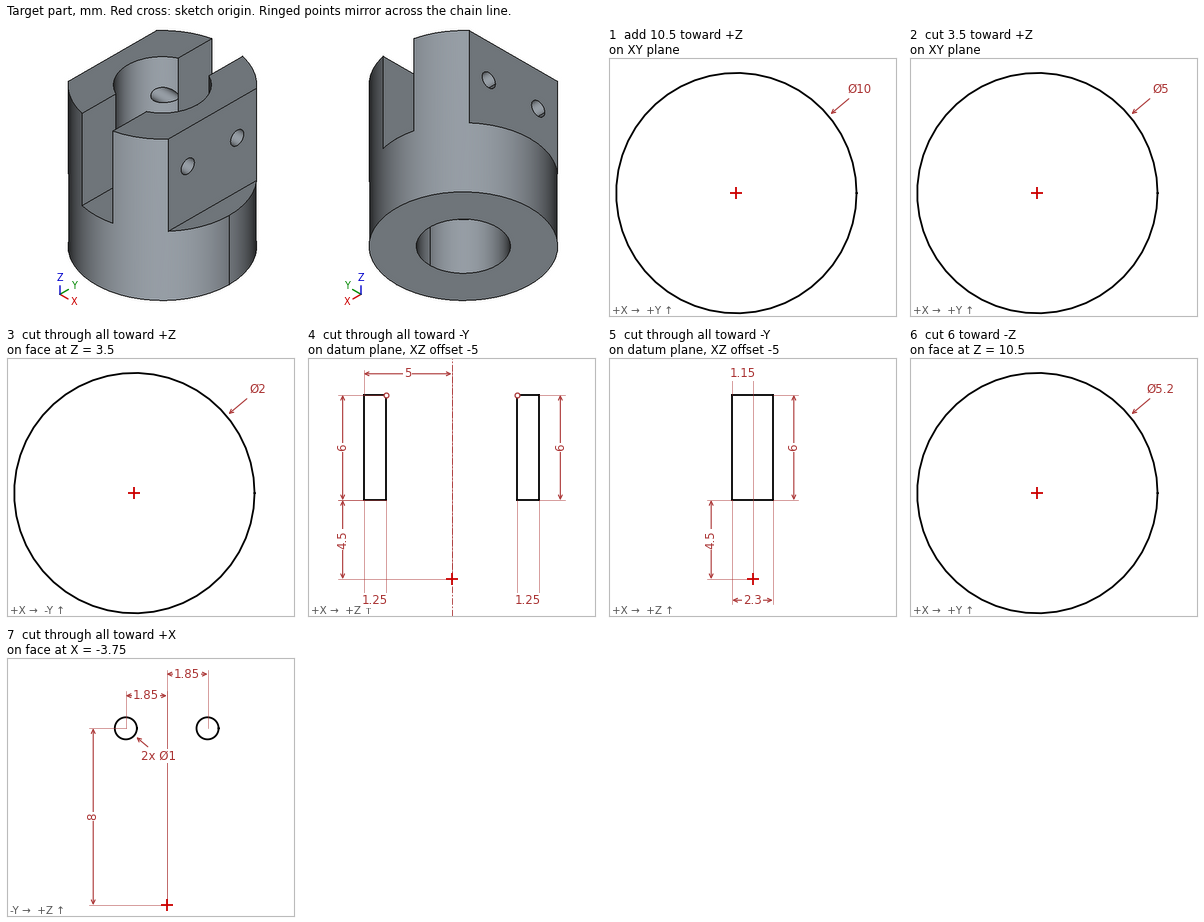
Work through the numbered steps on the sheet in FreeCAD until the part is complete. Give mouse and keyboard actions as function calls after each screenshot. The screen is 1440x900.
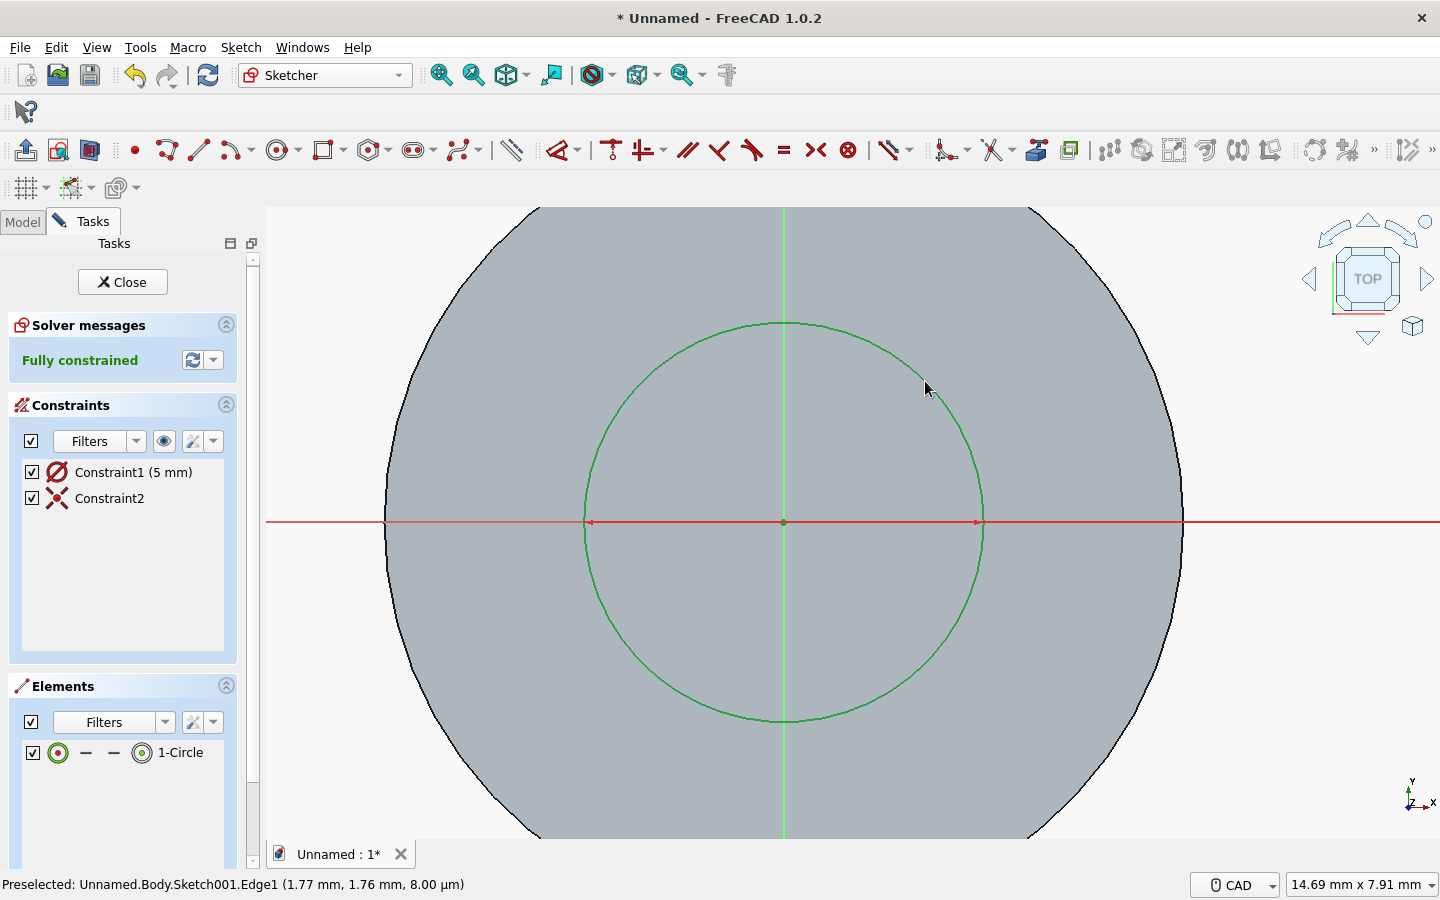
click(123, 282)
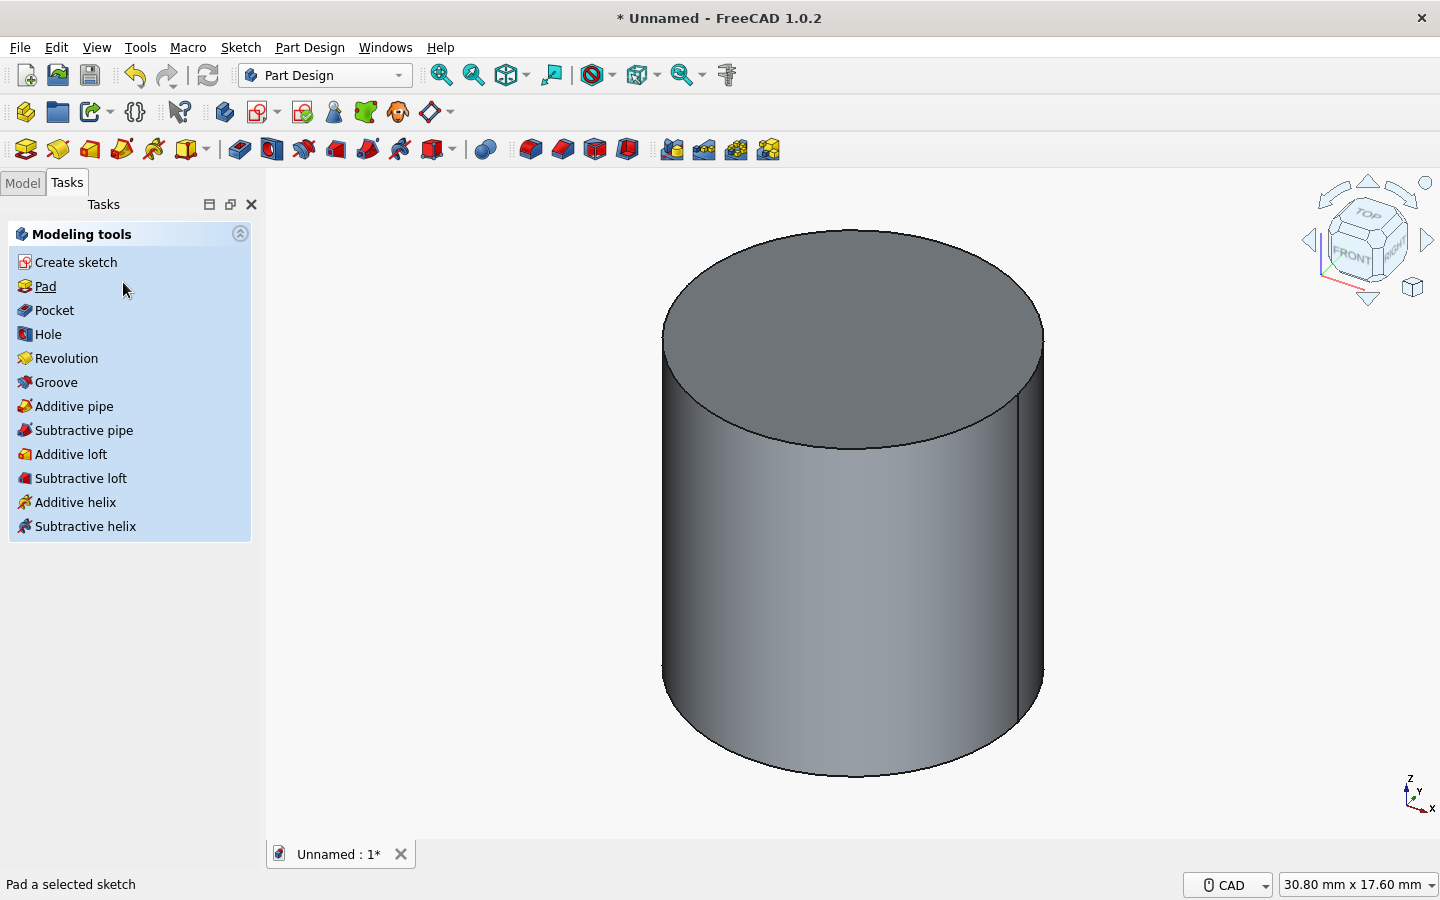
click(240, 150)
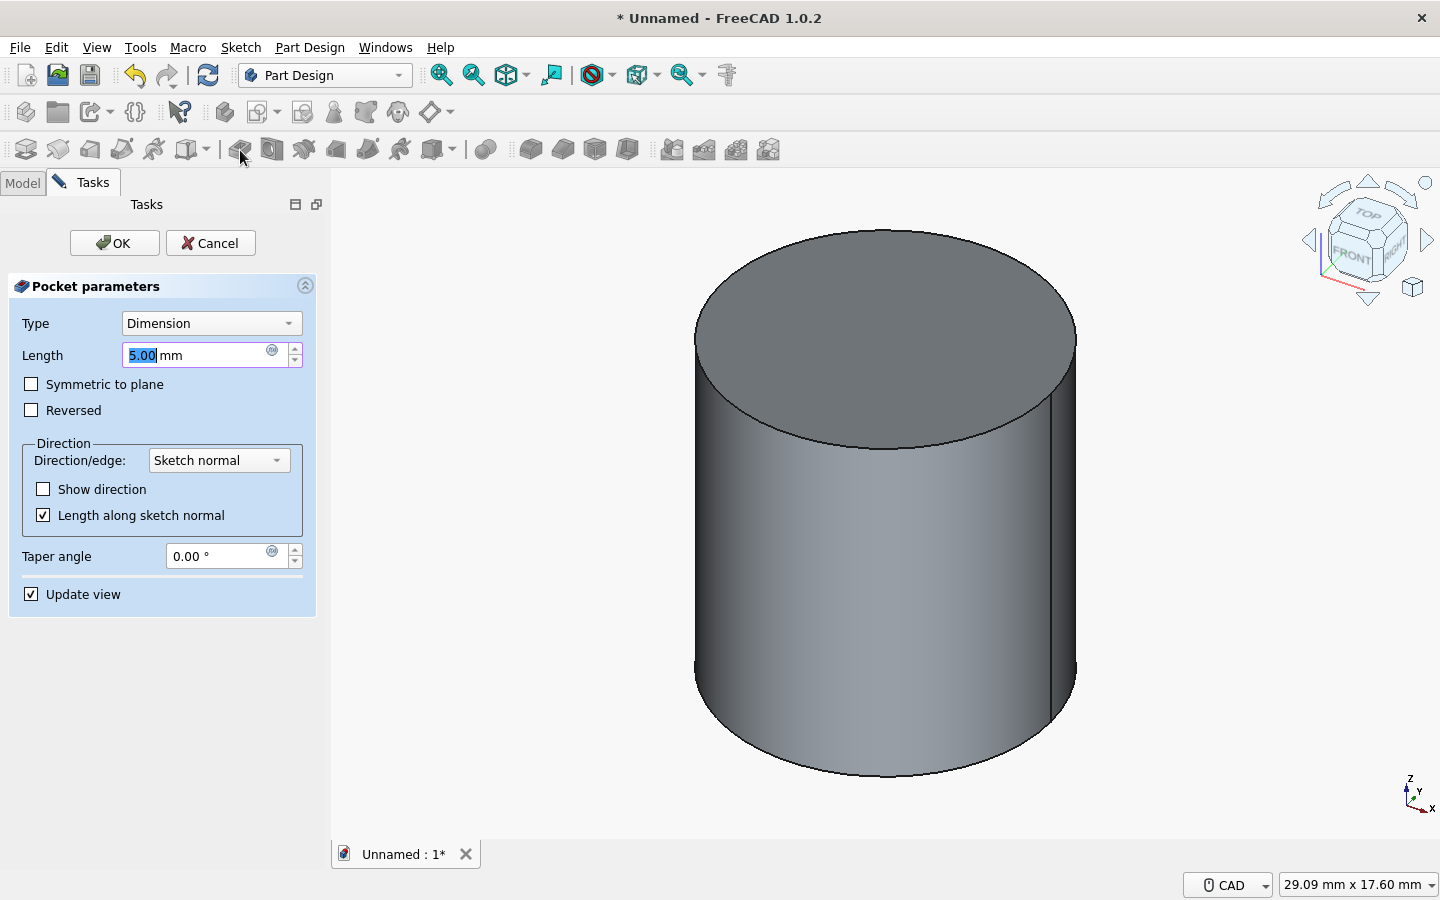
text(3.5)
key(Tab)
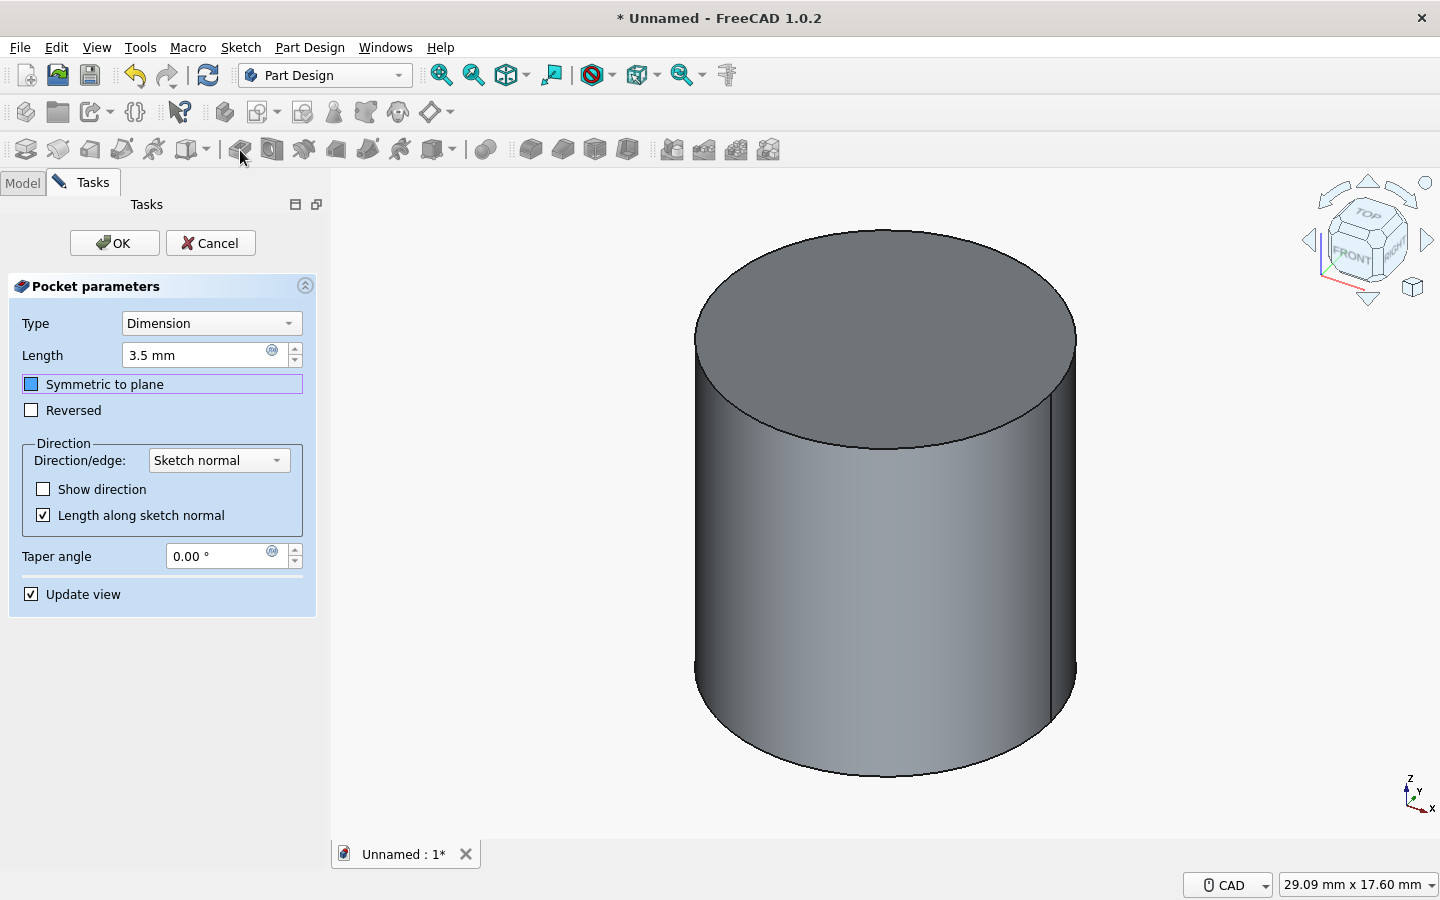
click(30, 410)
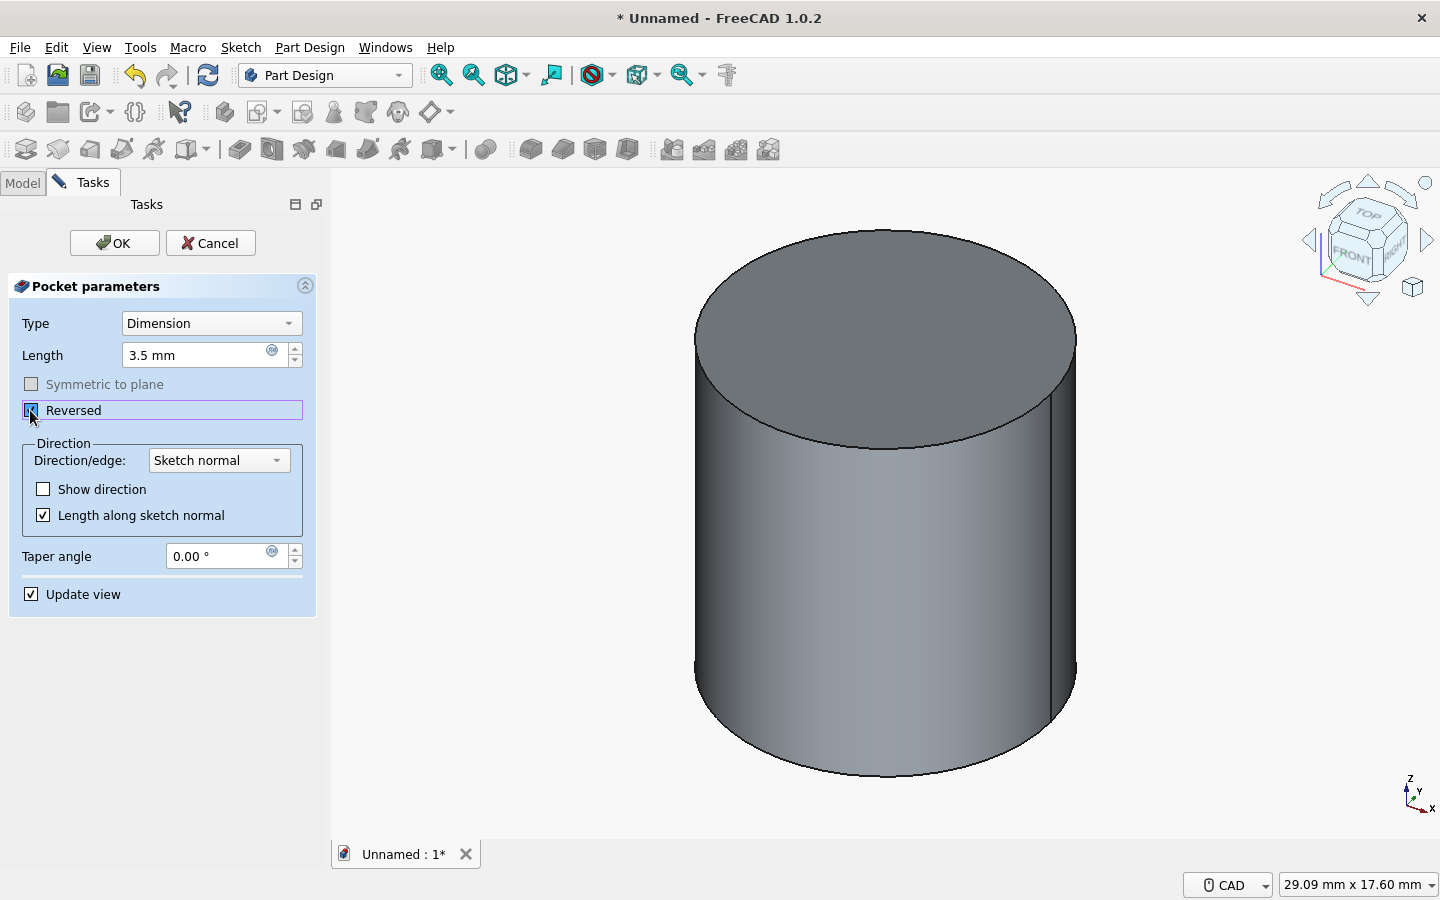
click(115, 243)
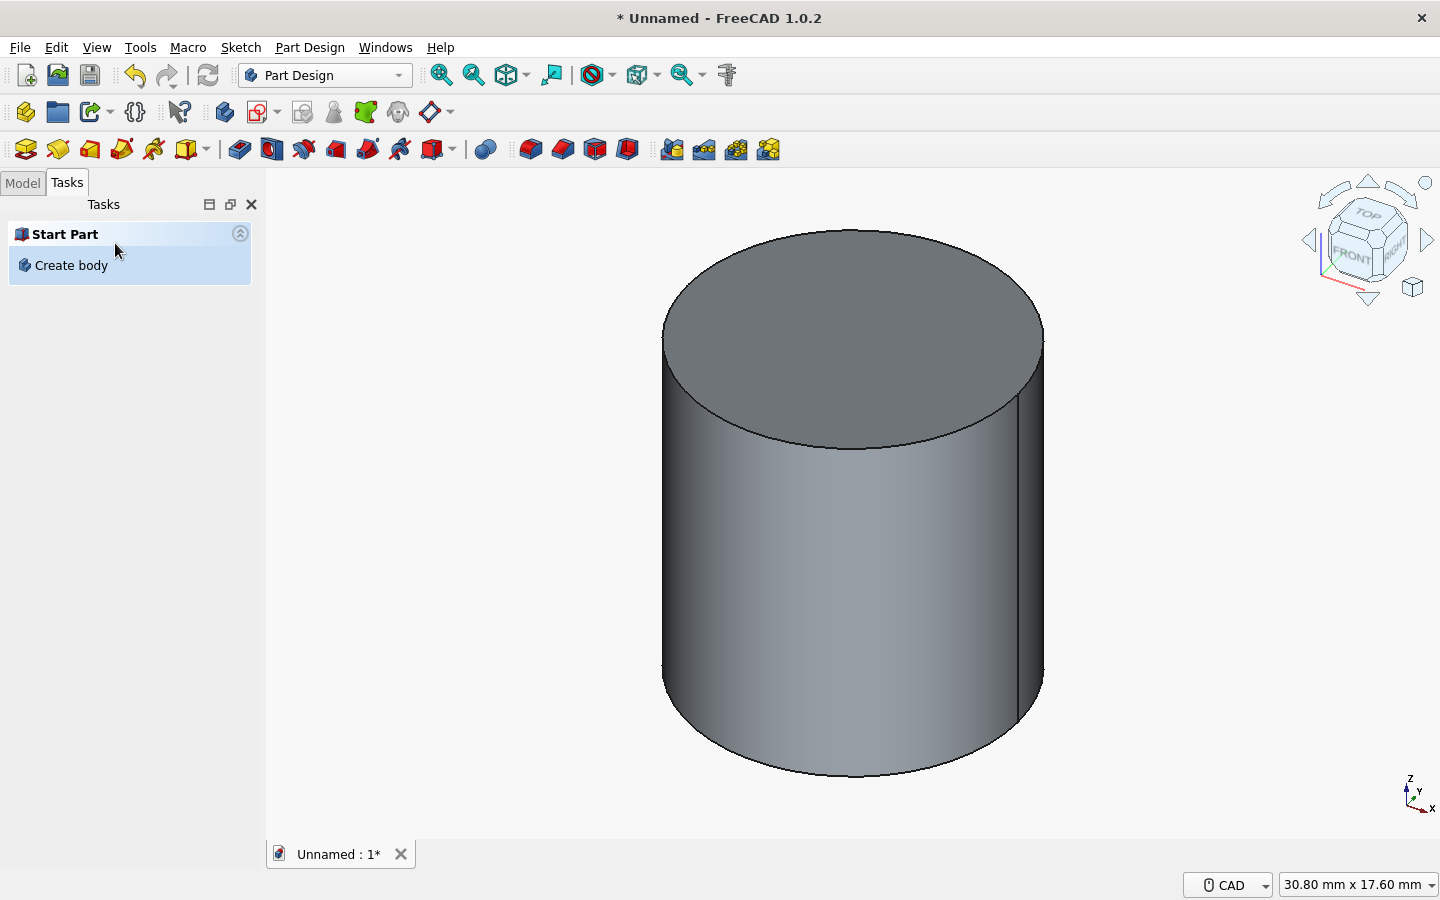
key(5)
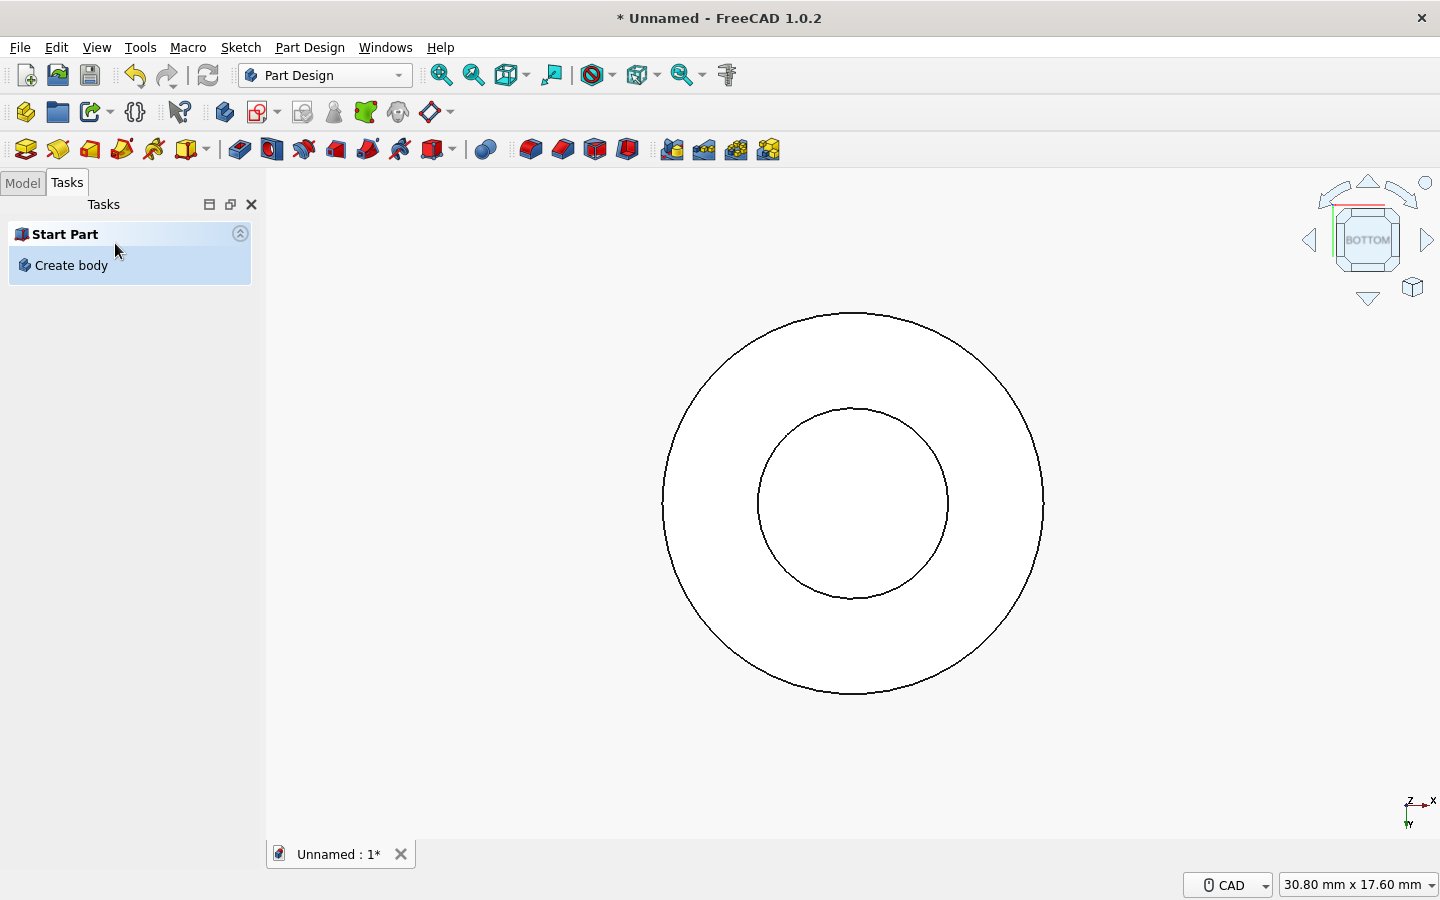
click(853, 502)